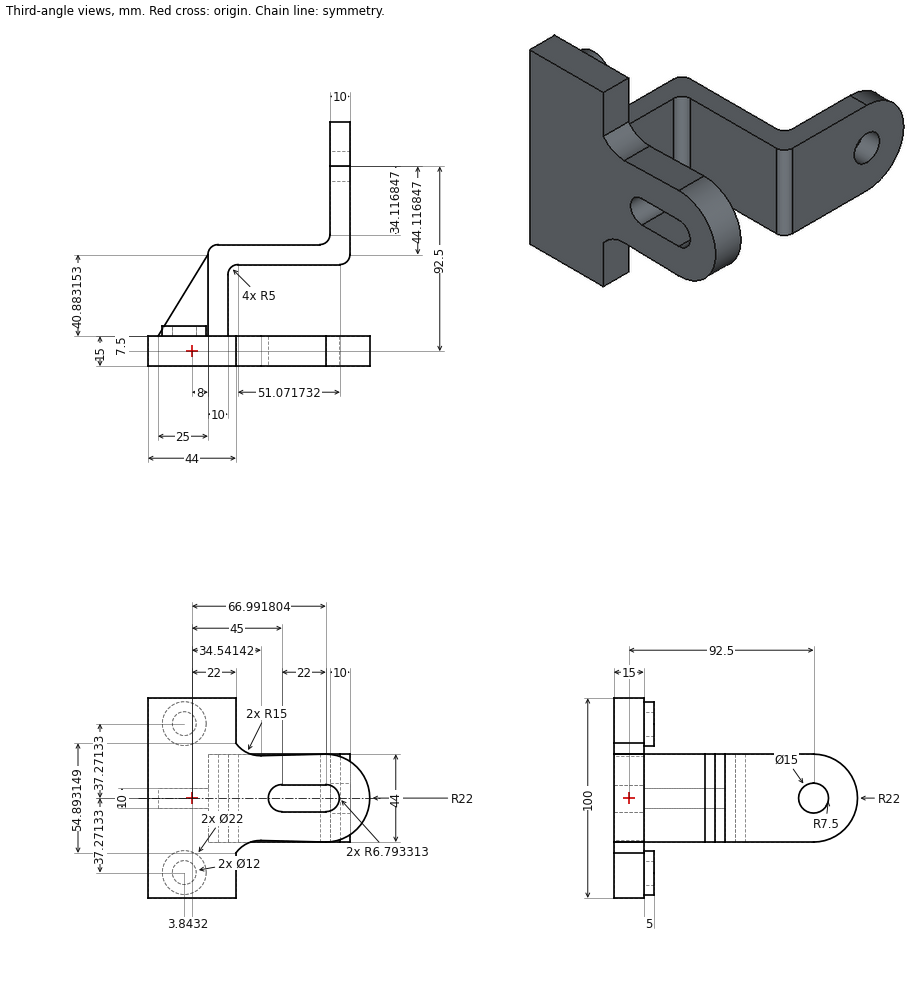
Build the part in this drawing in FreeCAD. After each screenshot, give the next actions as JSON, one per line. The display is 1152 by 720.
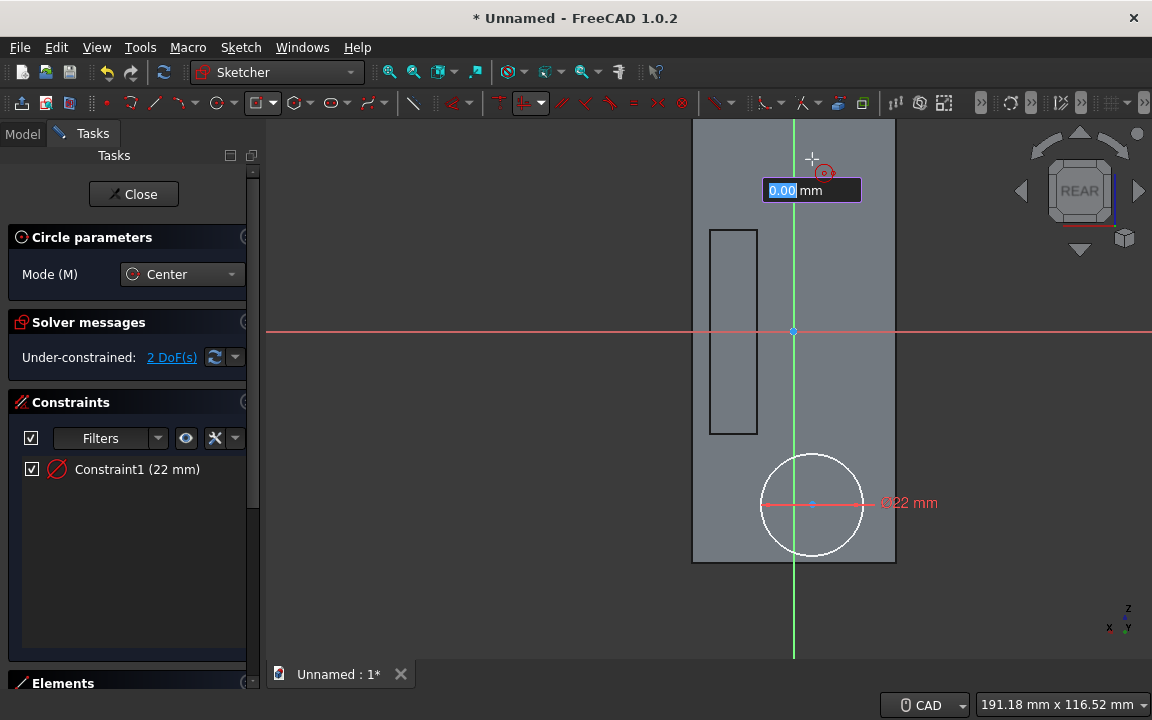
{"action": "scroll", "coordinate": [294, 631], "scroll_direction": "down", "scroll_amount": 1}
{"action": "mouse_move", "coordinate": [747, 215]}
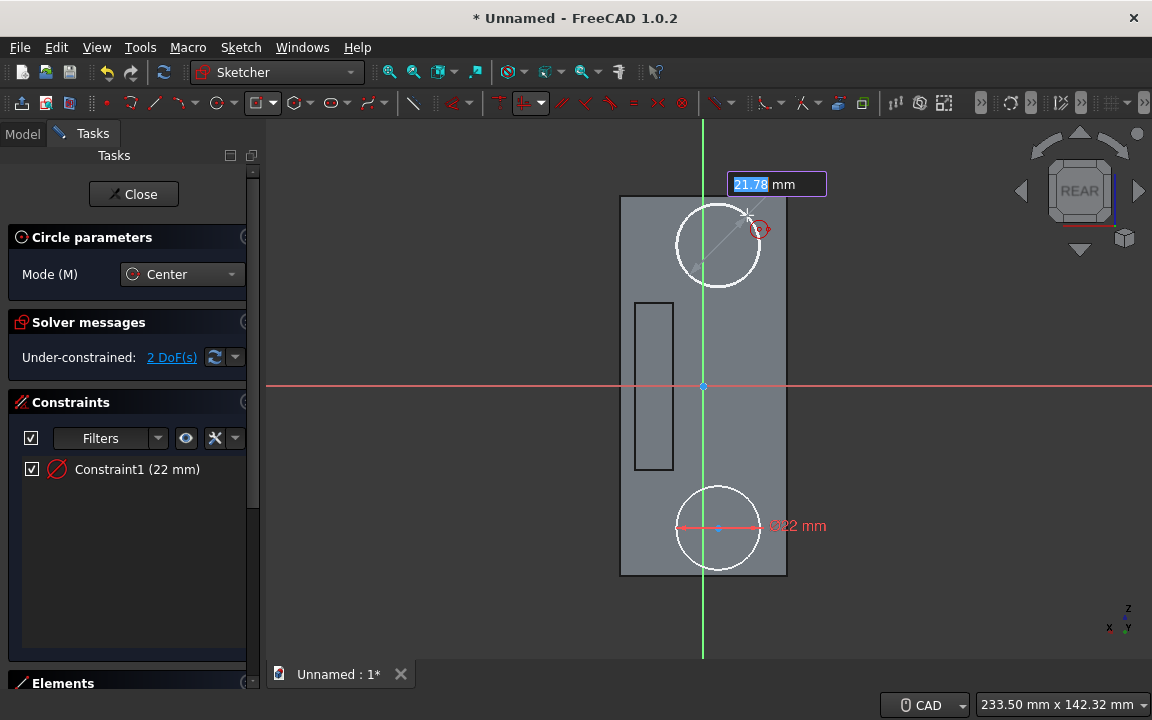
{"action": "type", "text": "22"}
{"action": "key", "text": "Return"}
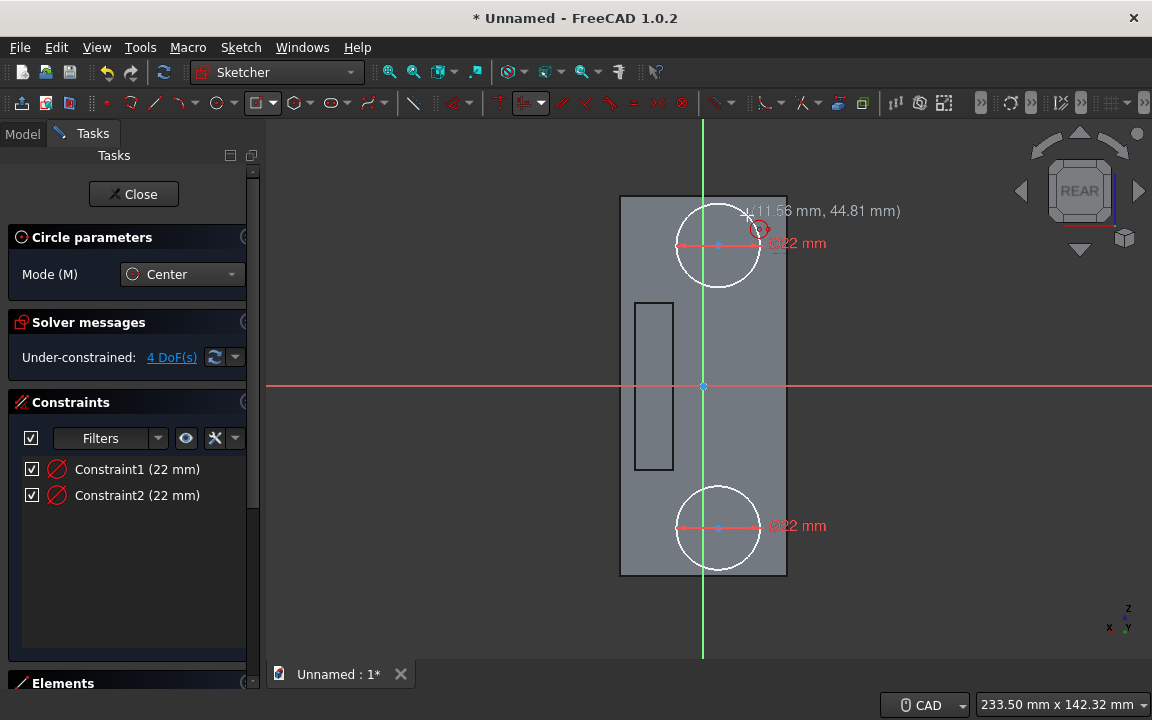
{"action": "left_click", "coordinate": [718, 528]}
{"action": "mouse_move", "coordinate": [734, 511]}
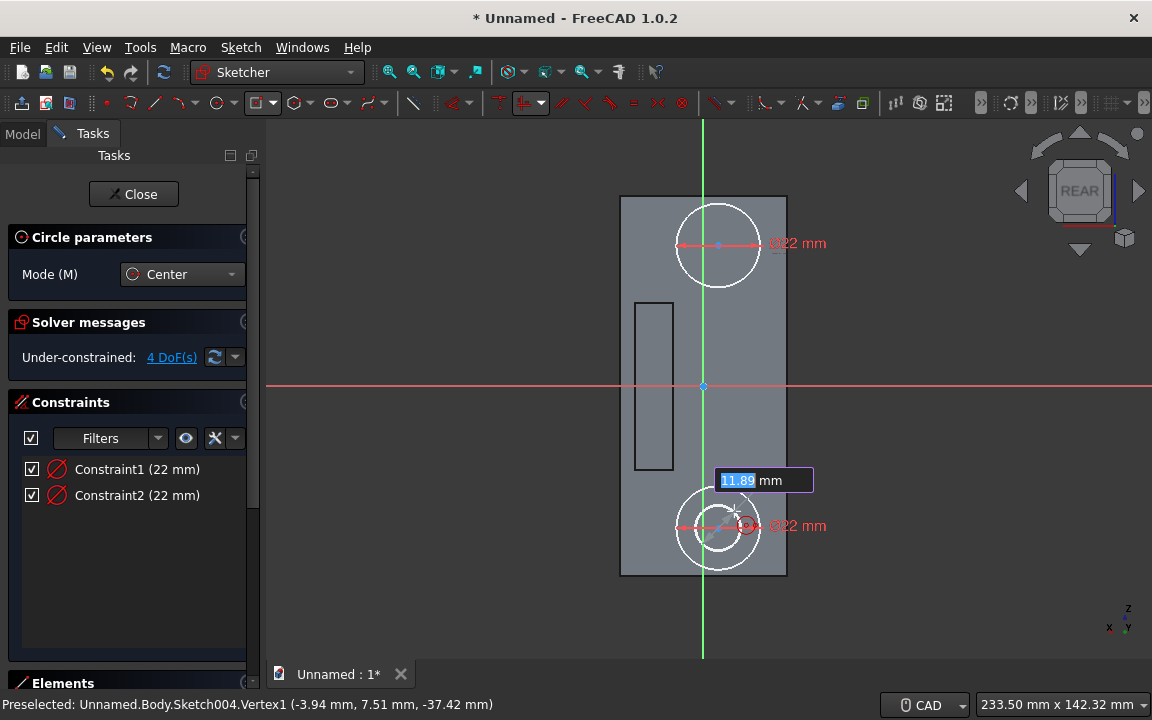
{"action": "type", "text": "12"}
{"action": "key", "text": "Return"}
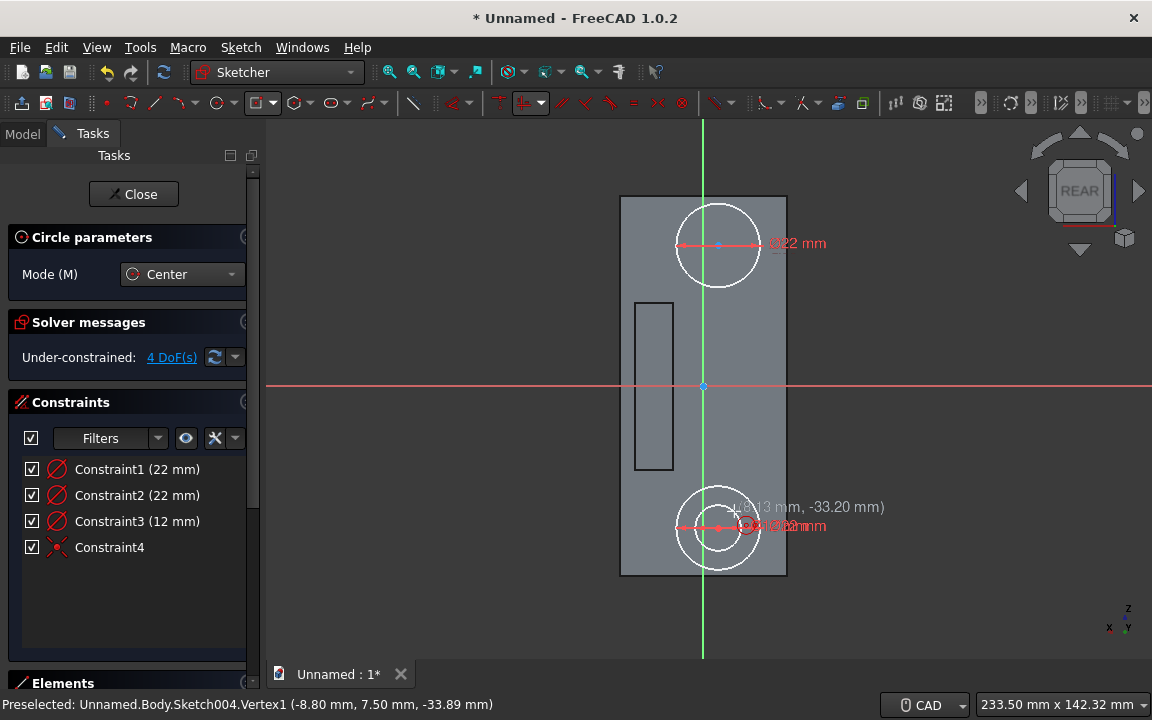
{"action": "left_click", "coordinate": [718, 246]}
{"action": "mouse_move", "coordinate": [734, 229]}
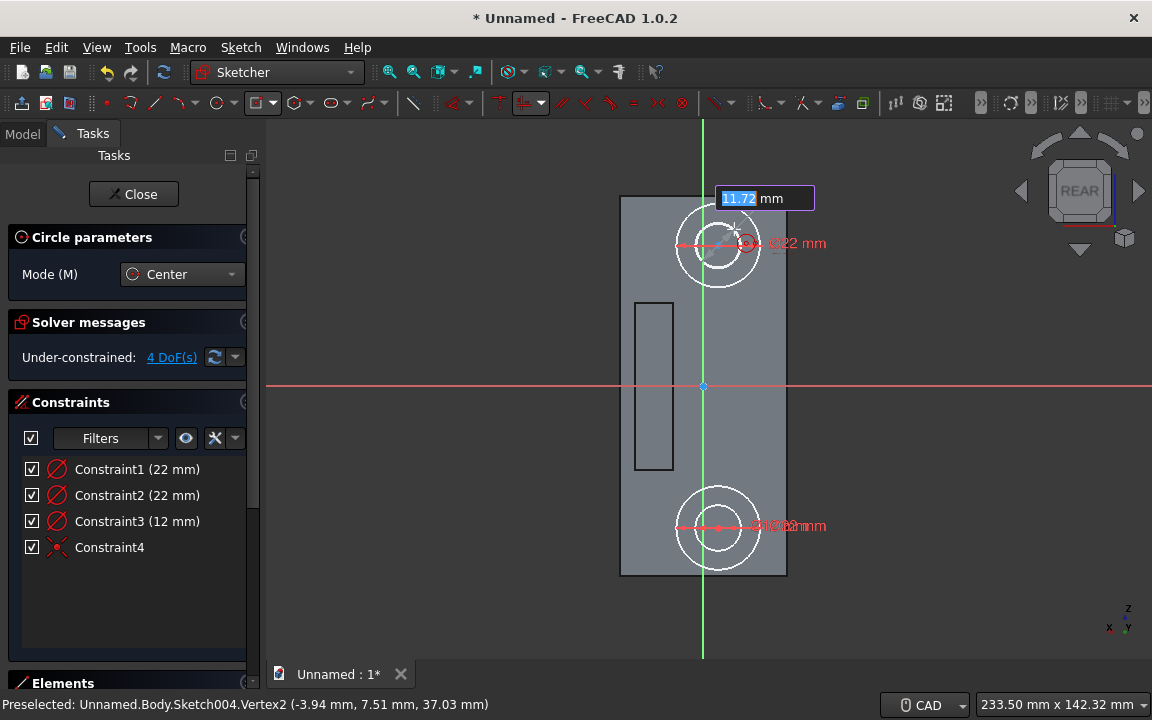
{"action": "type", "text": "12"}
{"action": "key", "text": "Return"}
{"action": "key", "text": "Escape"}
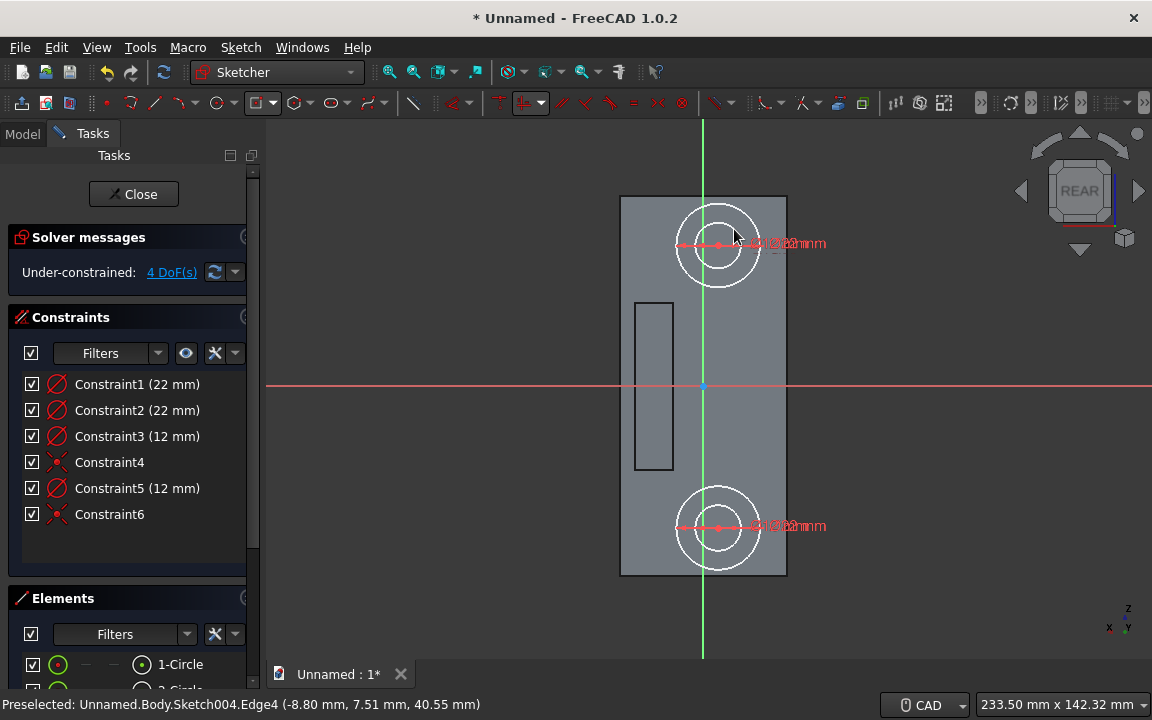
{"action": "left_click", "coordinate": [718, 528]}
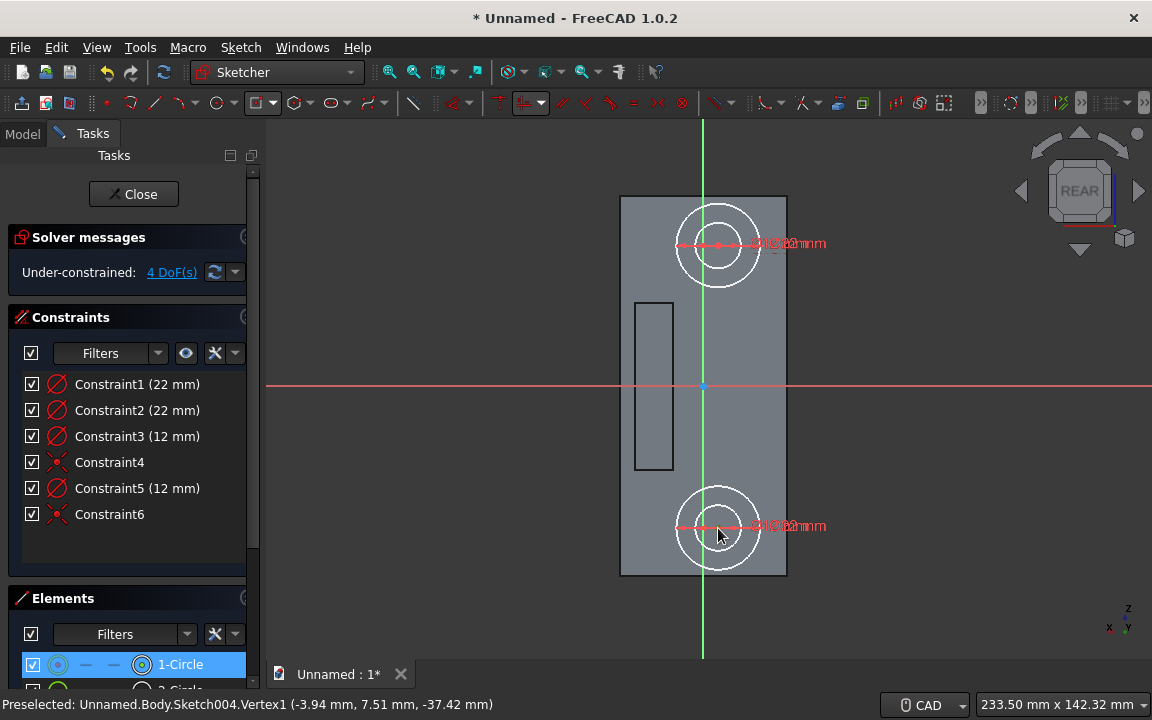
{"action": "left_click", "coordinate": [718, 246]}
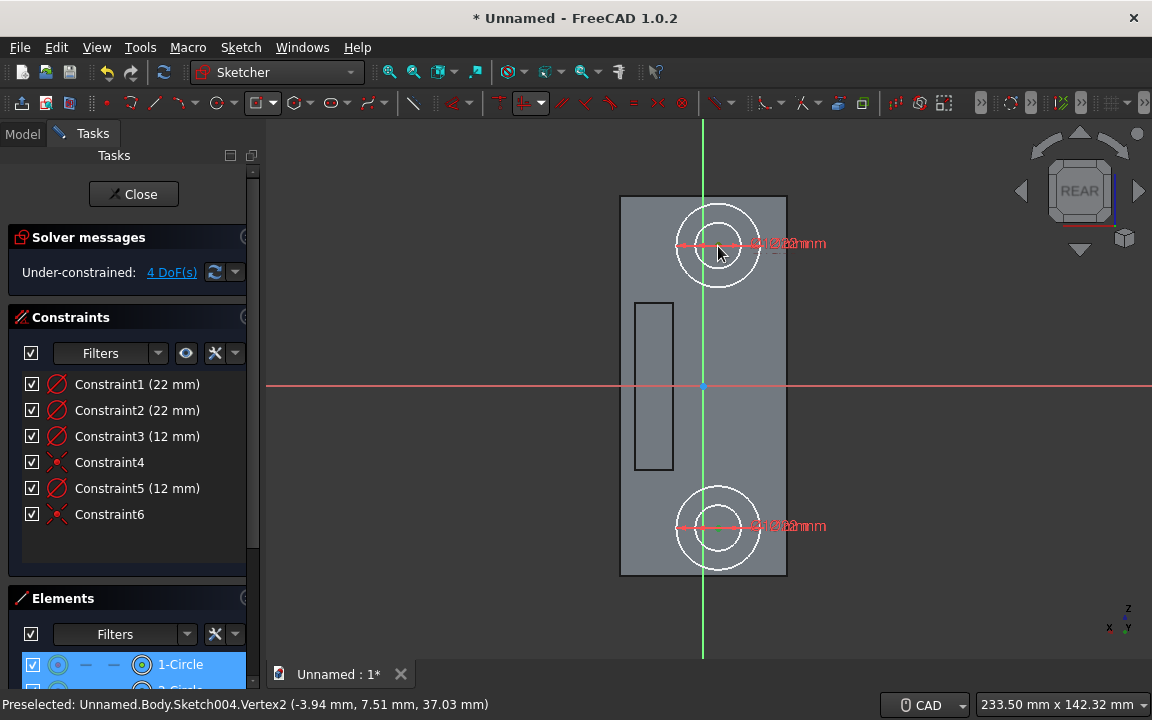
{"action": "key", "text": "v"}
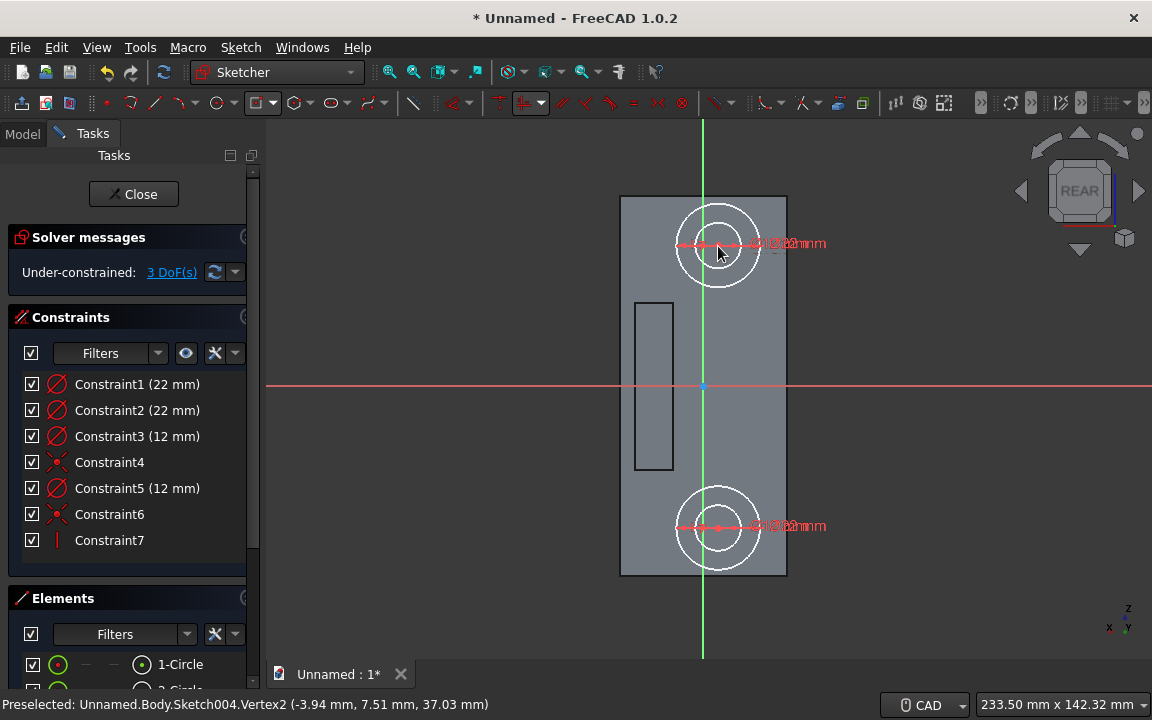
{"action": "left_click", "coordinate": [452, 104]}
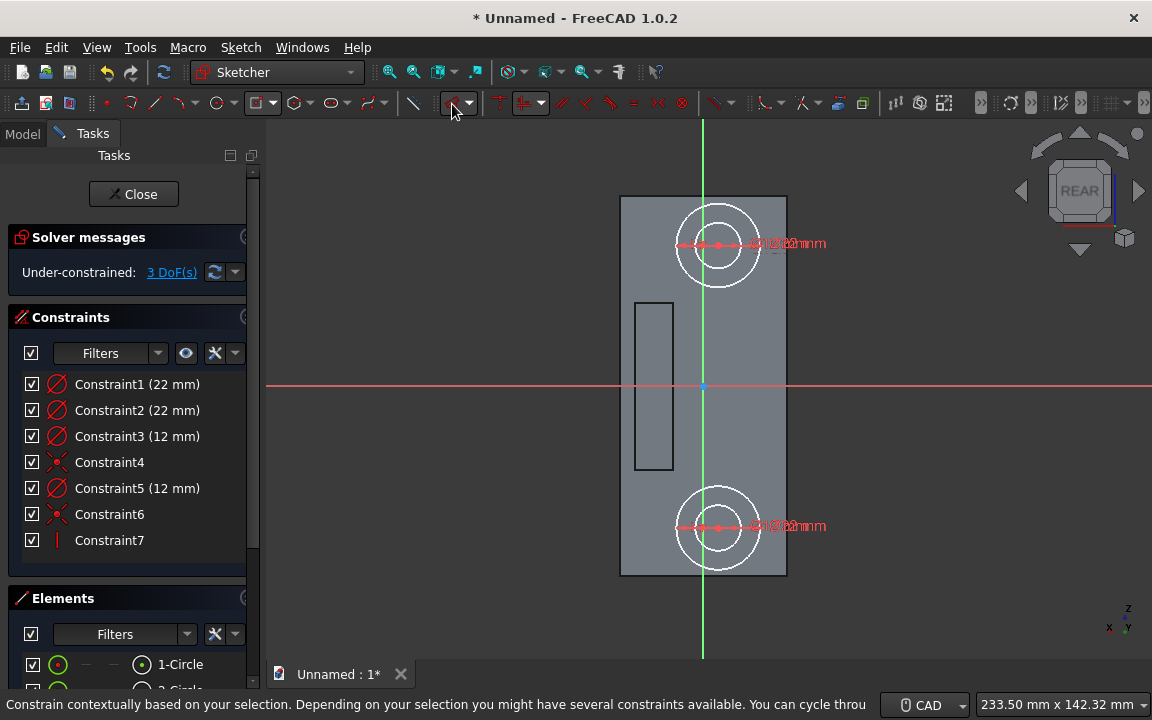
{"action": "scroll", "coordinate": [718, 528], "scroll_direction": "up", "scroll_amount": 6}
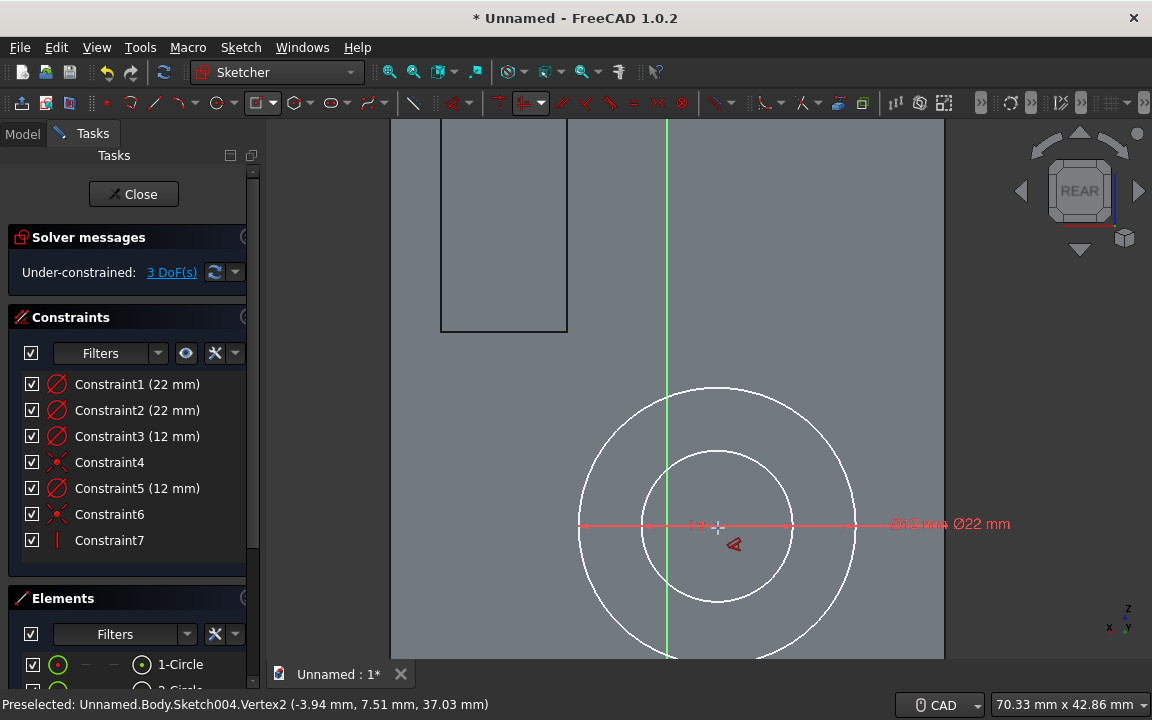
{"action": "left_click", "coordinate": [717, 526]}
{"action": "left_click", "coordinate": [692, 560]}